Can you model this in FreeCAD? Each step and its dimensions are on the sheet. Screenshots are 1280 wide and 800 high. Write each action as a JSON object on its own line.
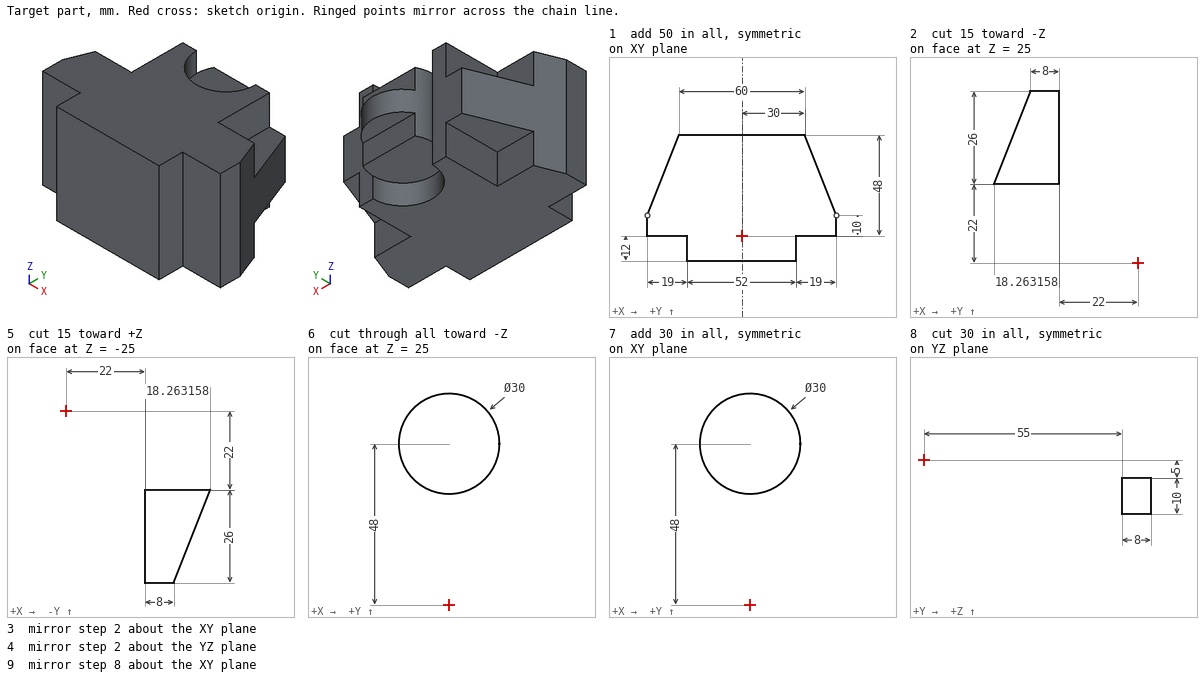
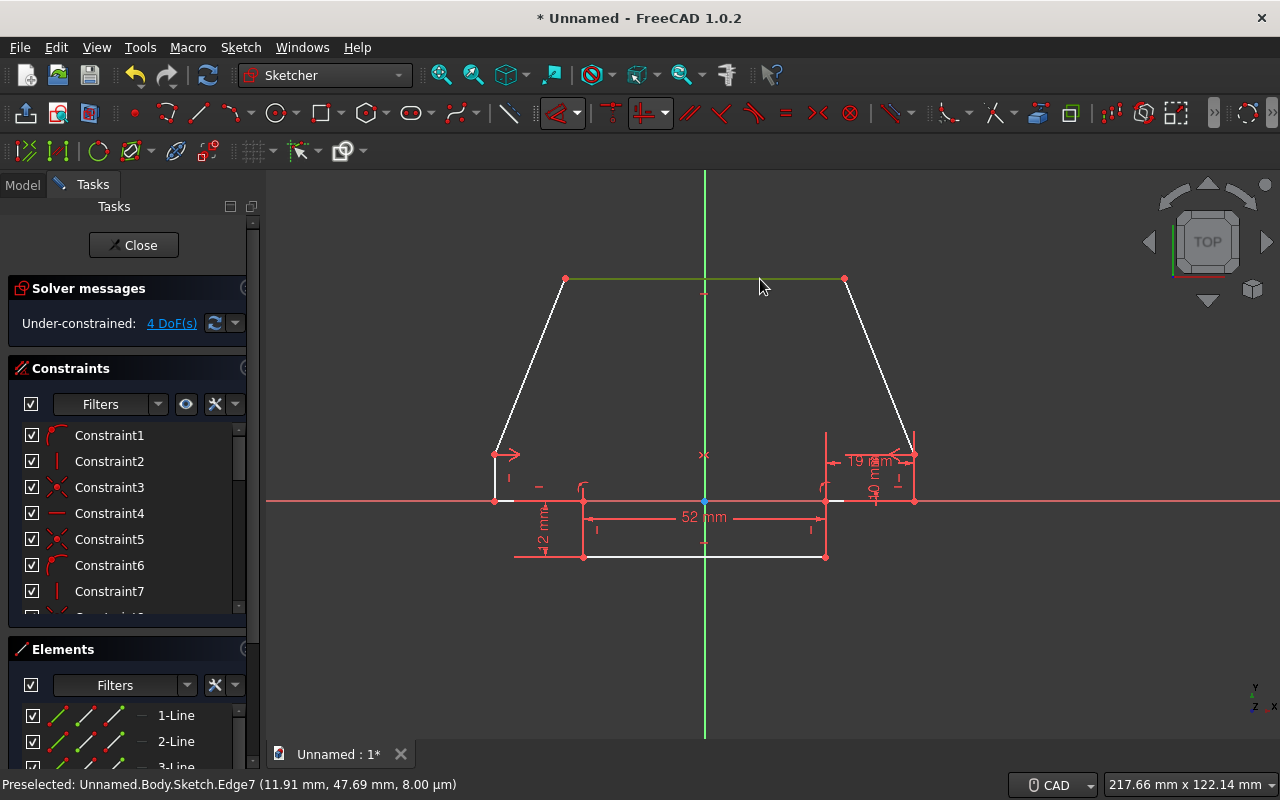
{"action": "left_click", "coordinate": [580, 114]}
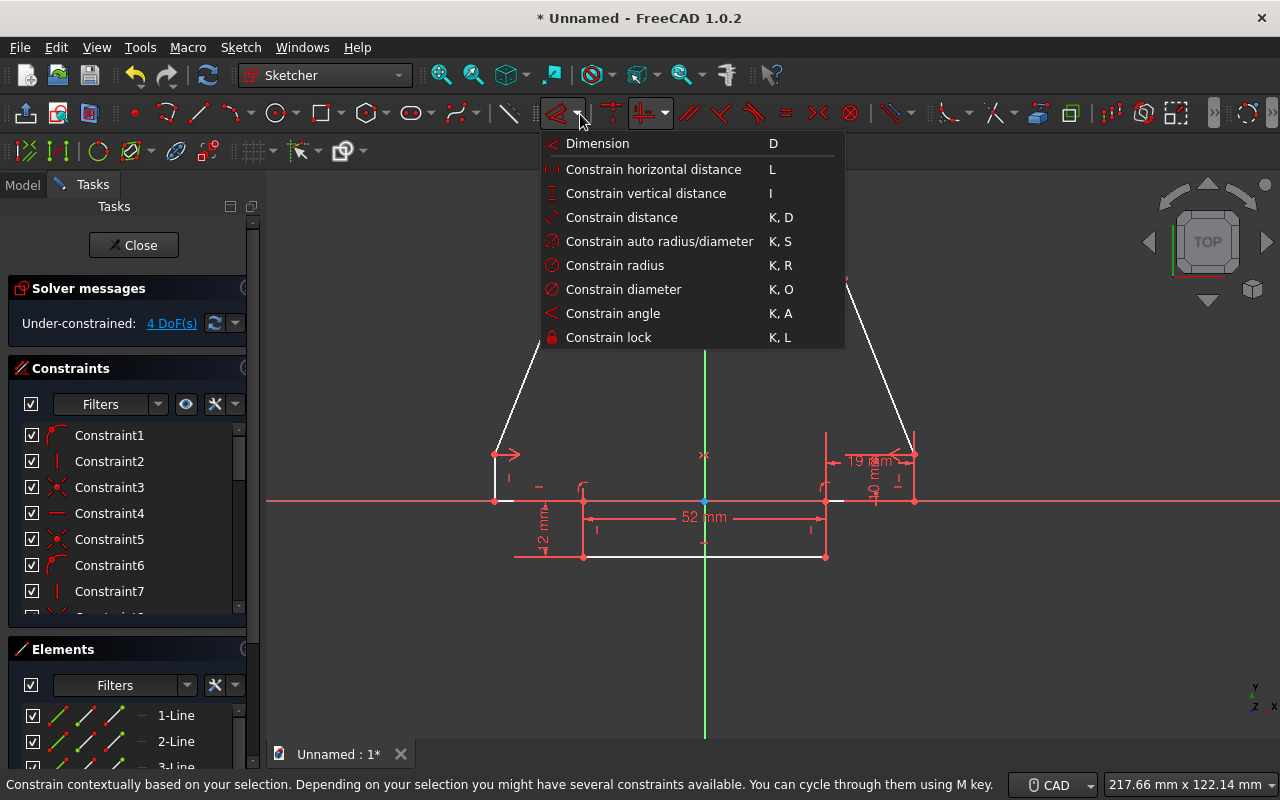
{"action": "left_click", "coordinate": [693, 169]}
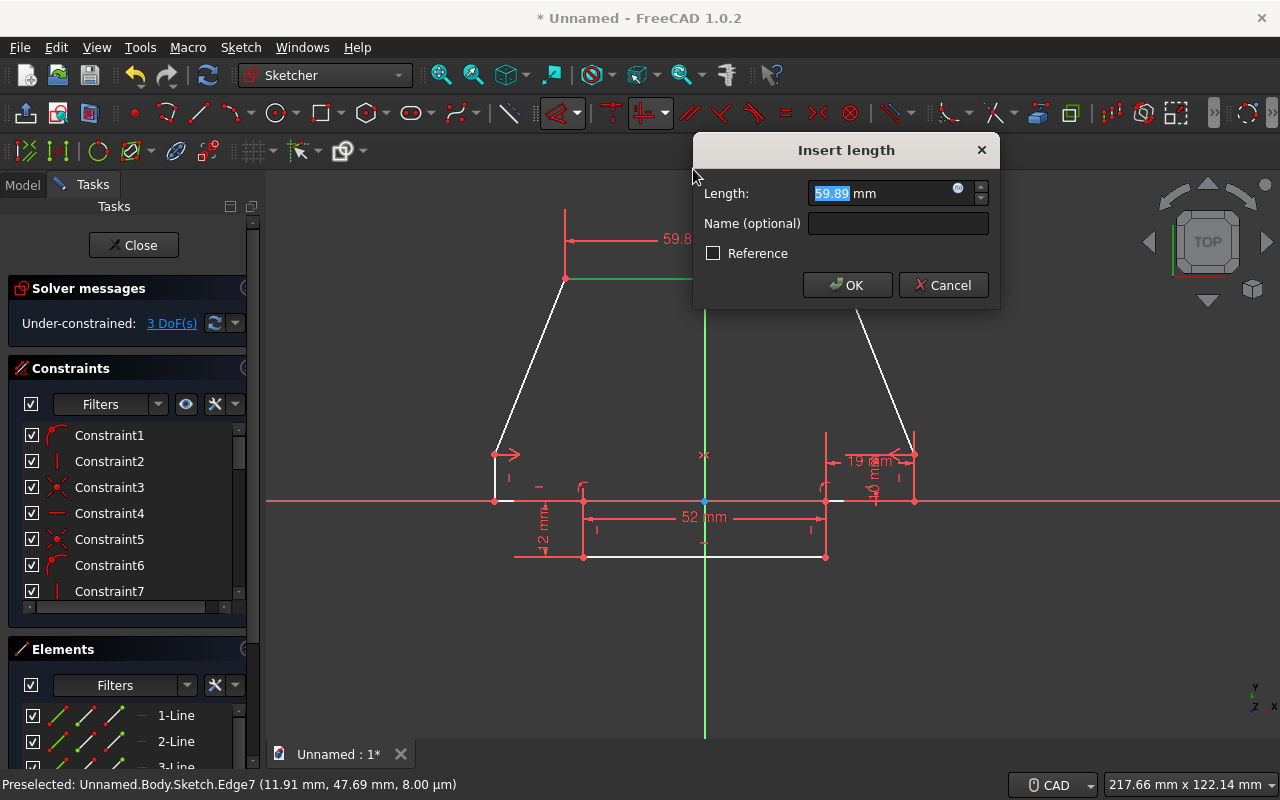
{"action": "type", "text": "60"}
{"action": "key", "text": "Return"}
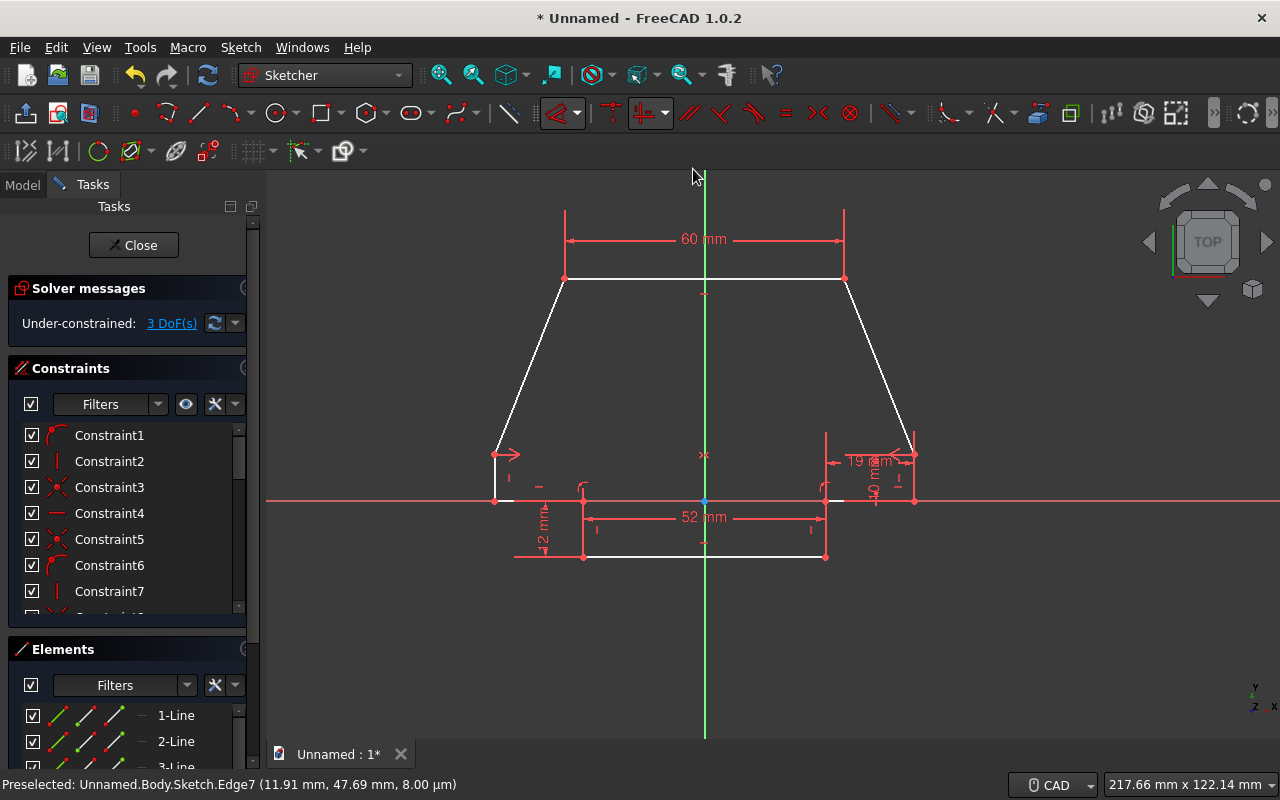
{"action": "left_click", "coordinate": [521, 501]}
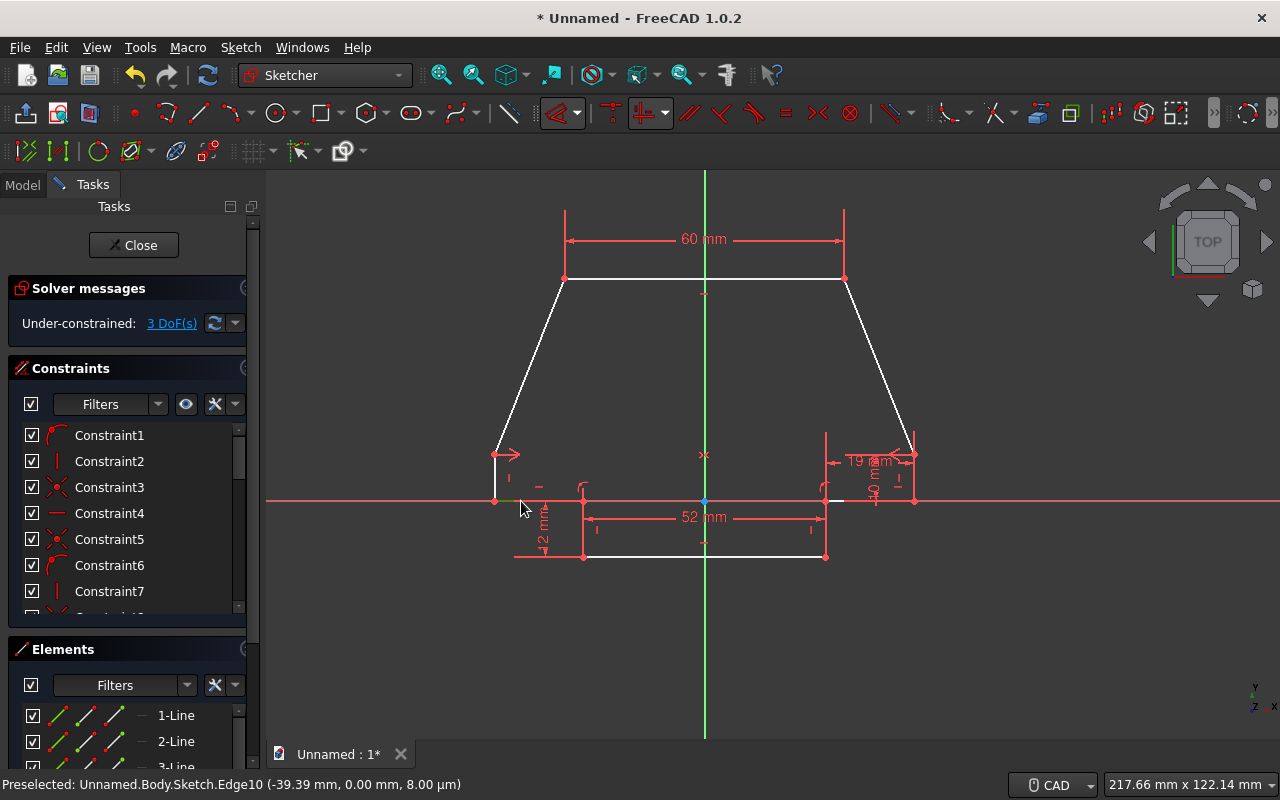
{"action": "key", "text": "l"}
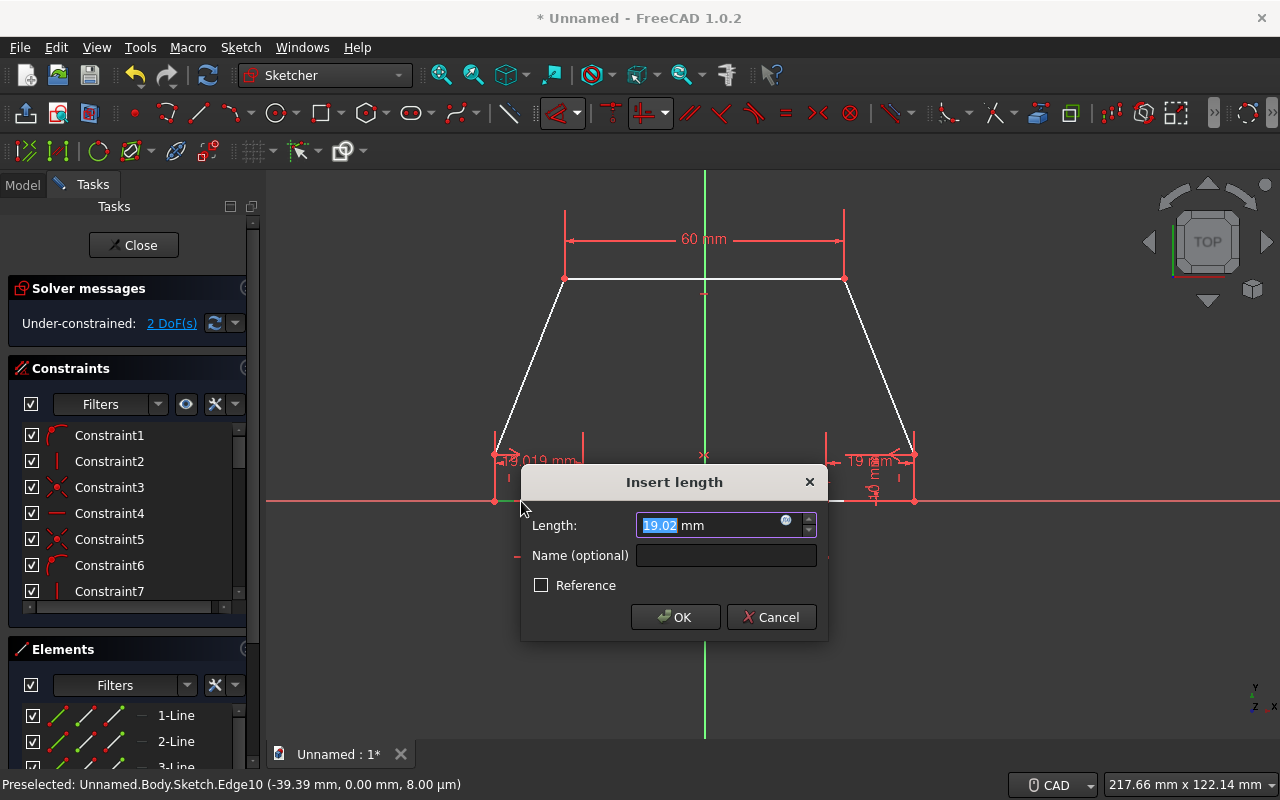
{"action": "type", "text": "19"}
{"action": "key", "text": "Return"}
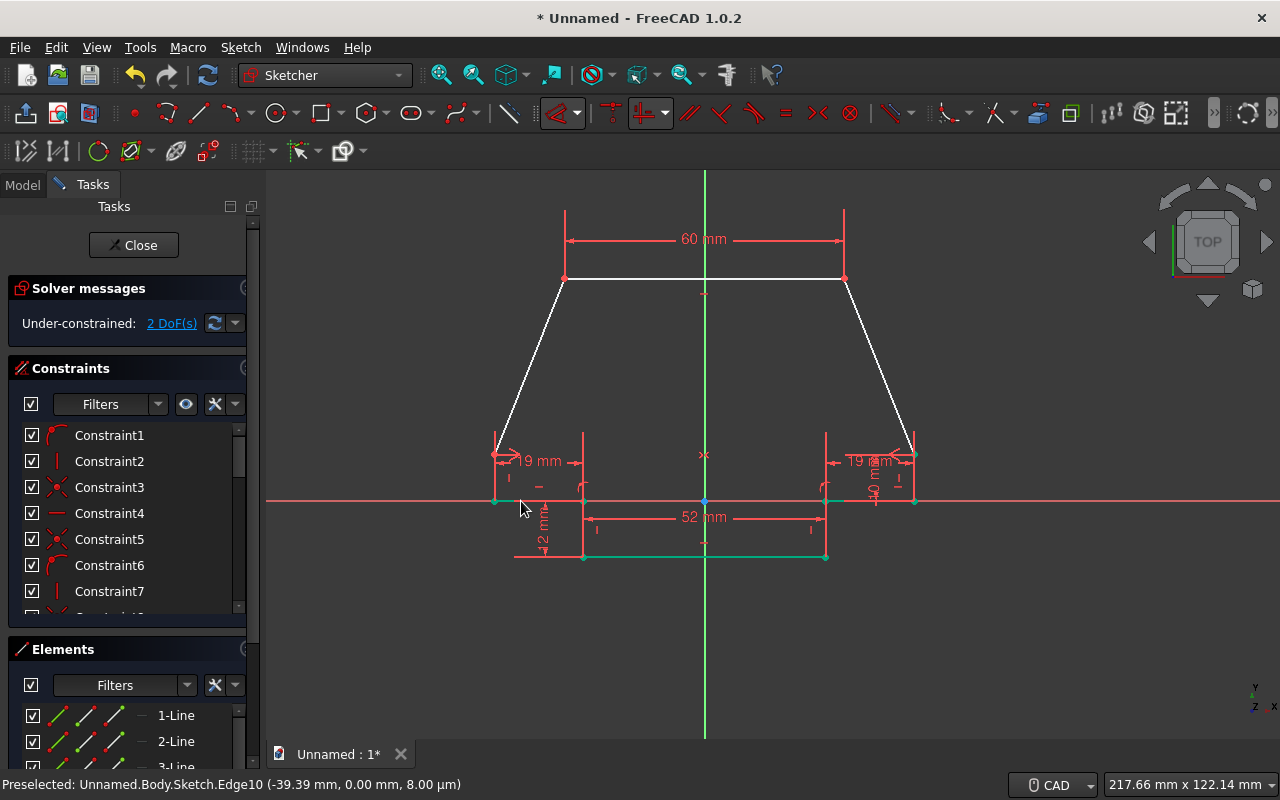
{"action": "left_click", "coordinate": [844, 279]}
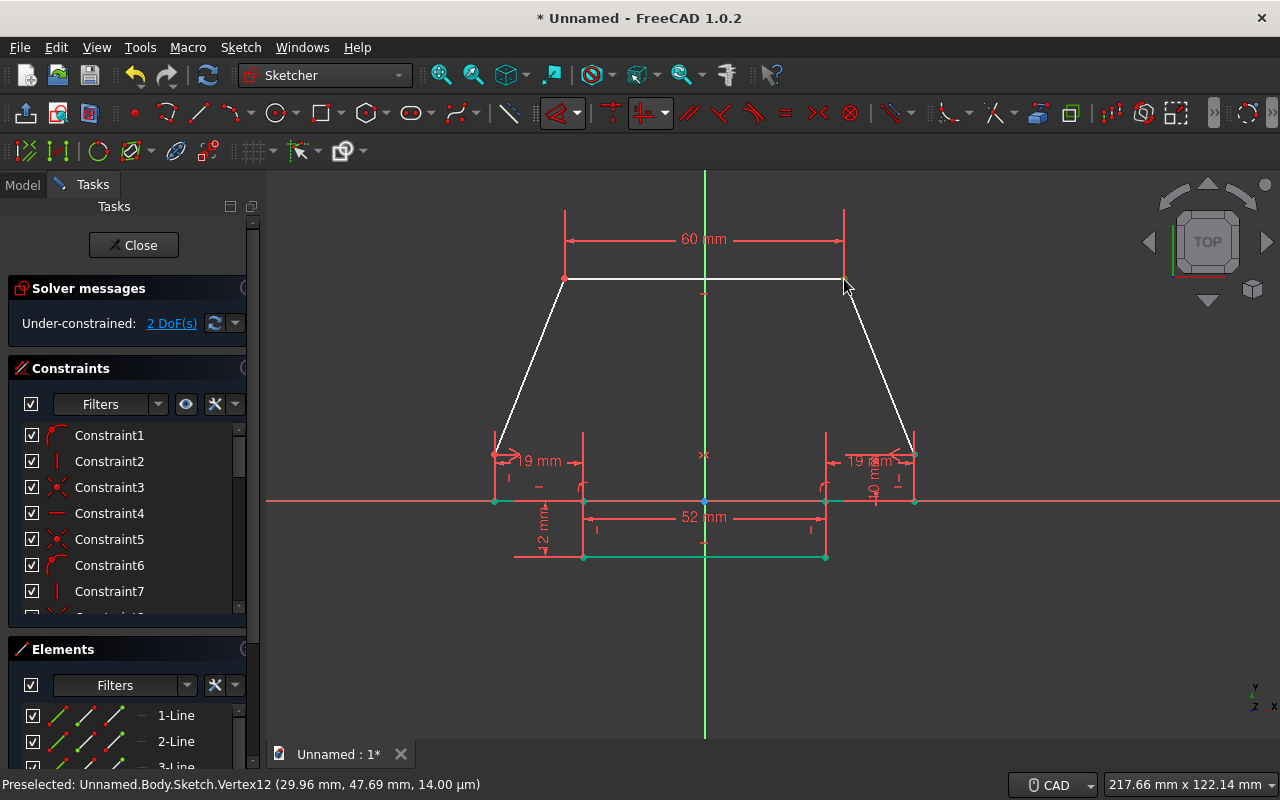
{"action": "key", "text": "l"}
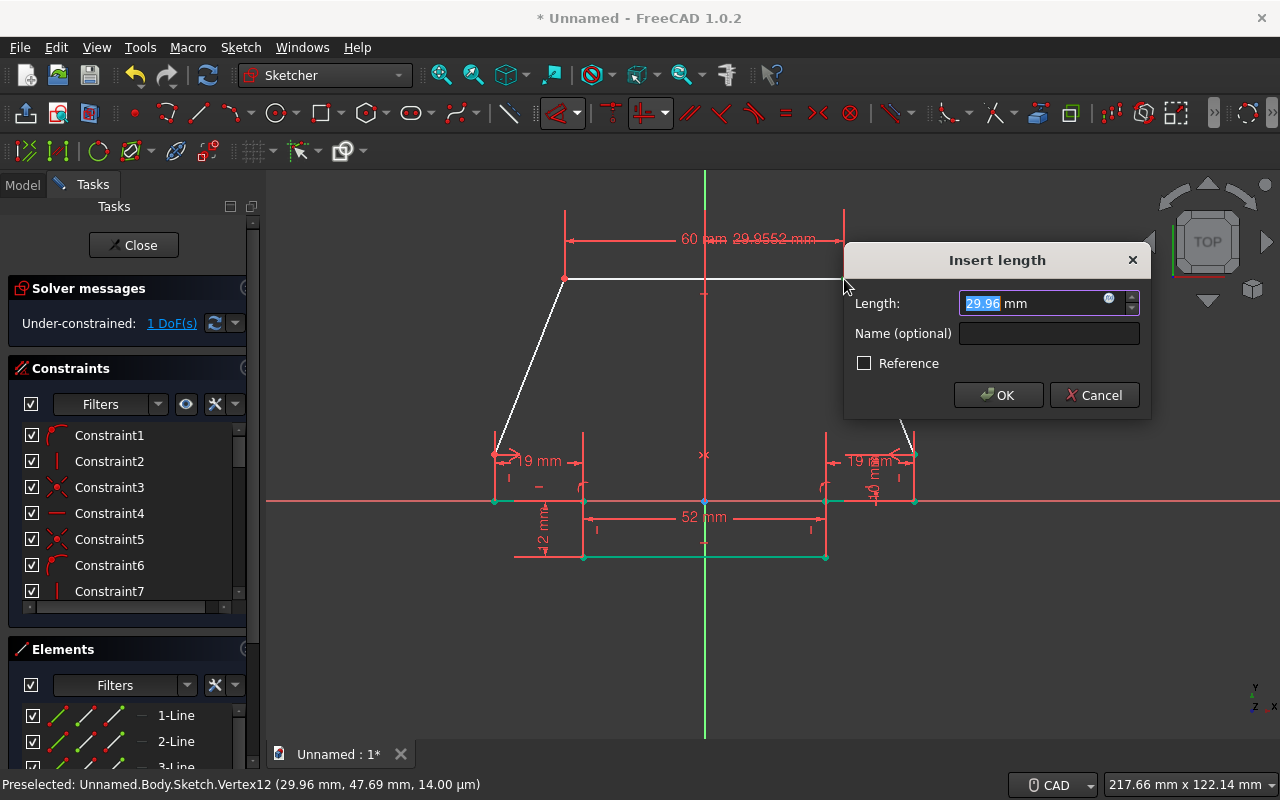
{"action": "type", "text": "30"}
{"action": "key", "text": "Return"}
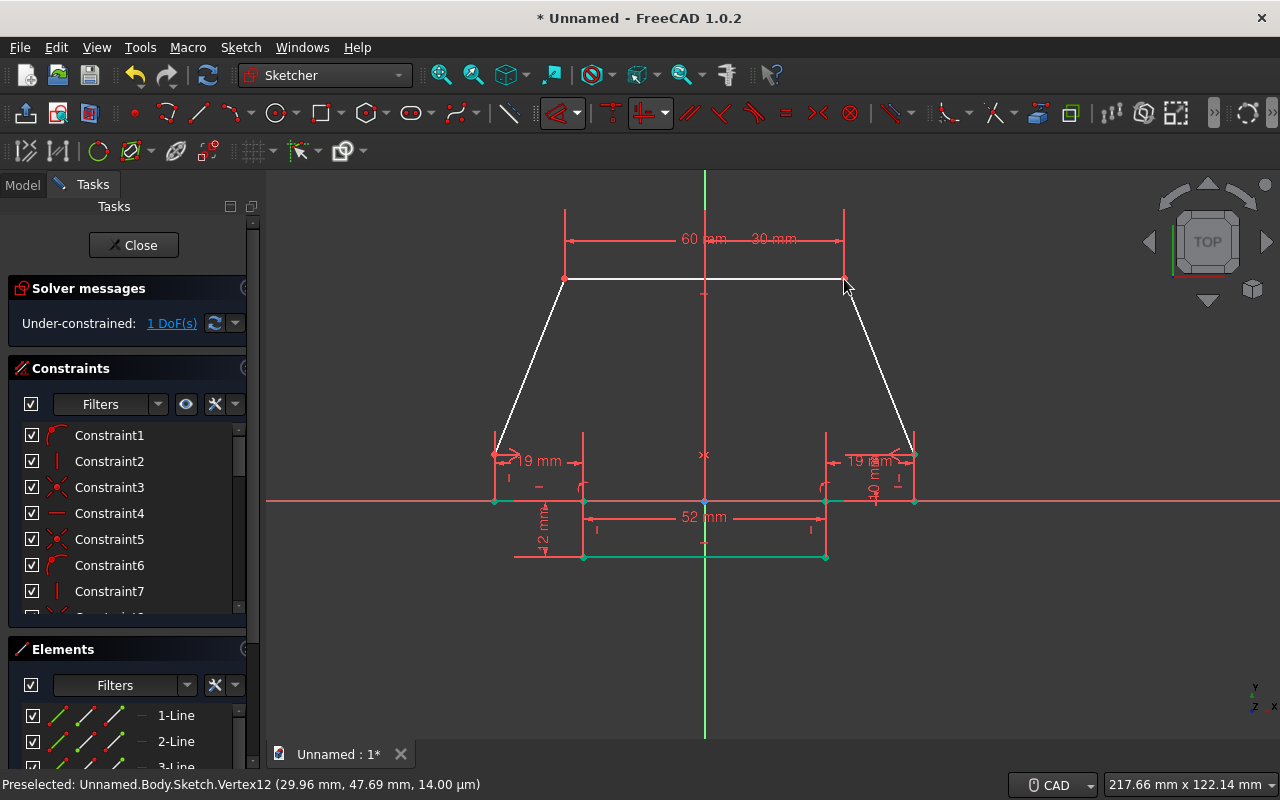
{"action": "left_click", "coordinate": [844, 279]}